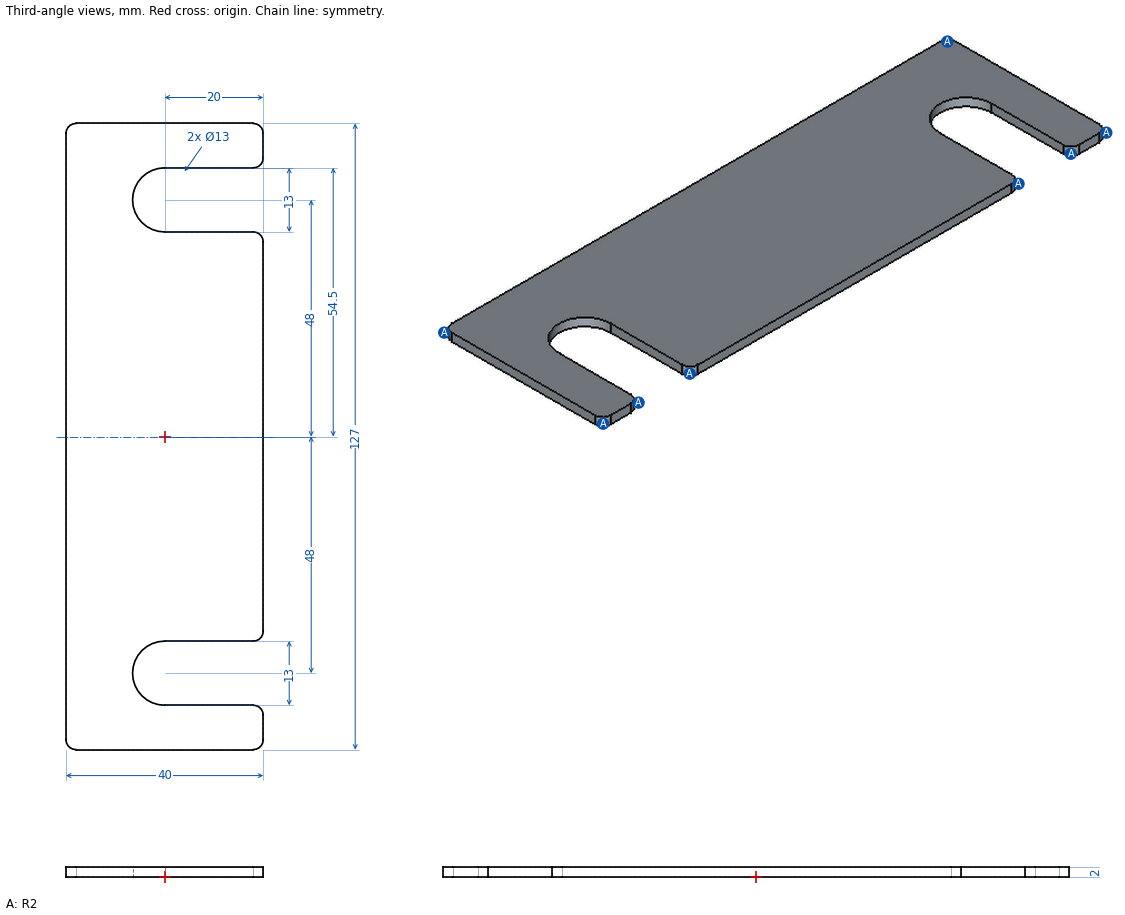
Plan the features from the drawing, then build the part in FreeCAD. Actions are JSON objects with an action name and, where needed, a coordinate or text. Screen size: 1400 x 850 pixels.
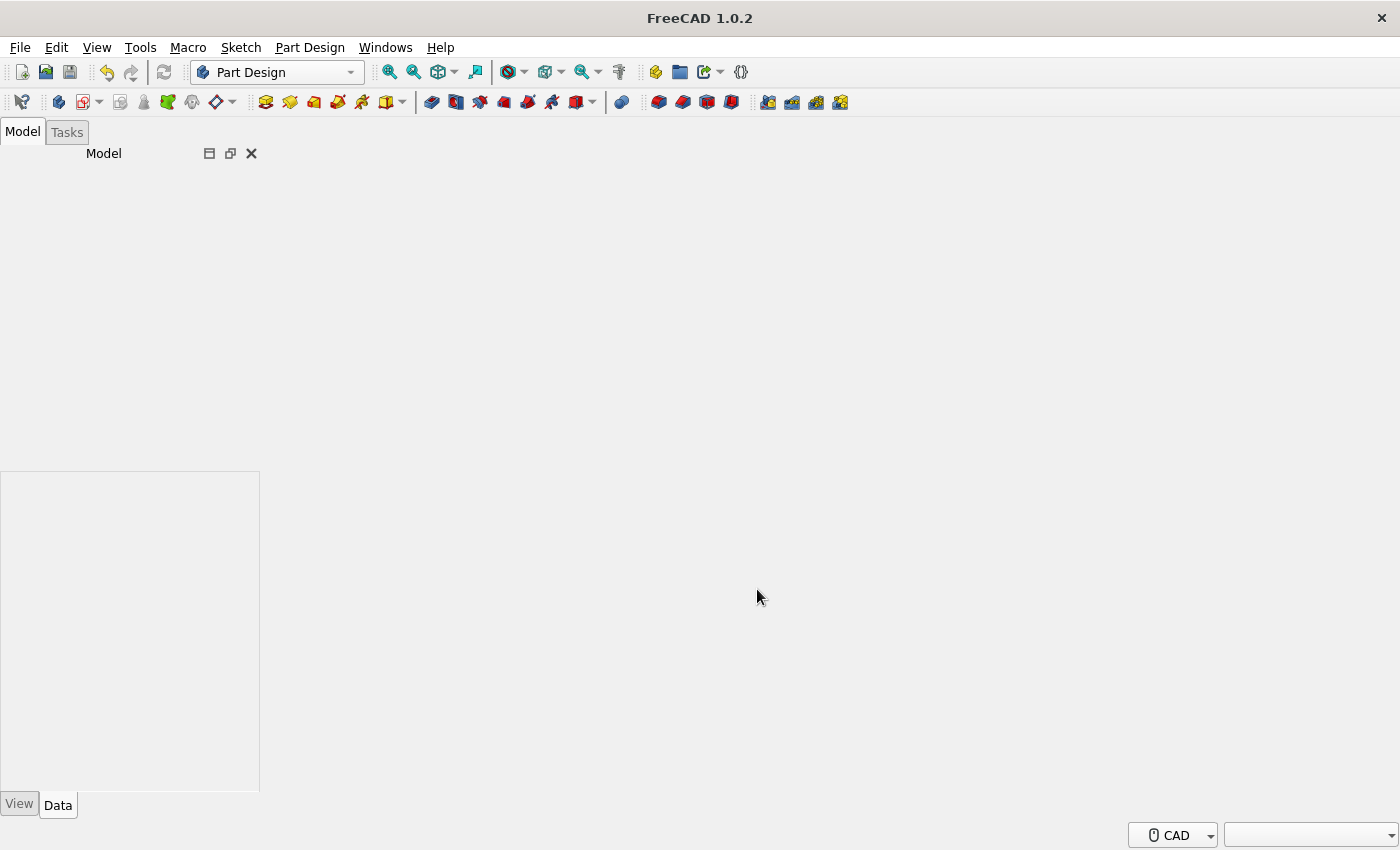
{"action": "left_click", "coordinate": [22, 72]}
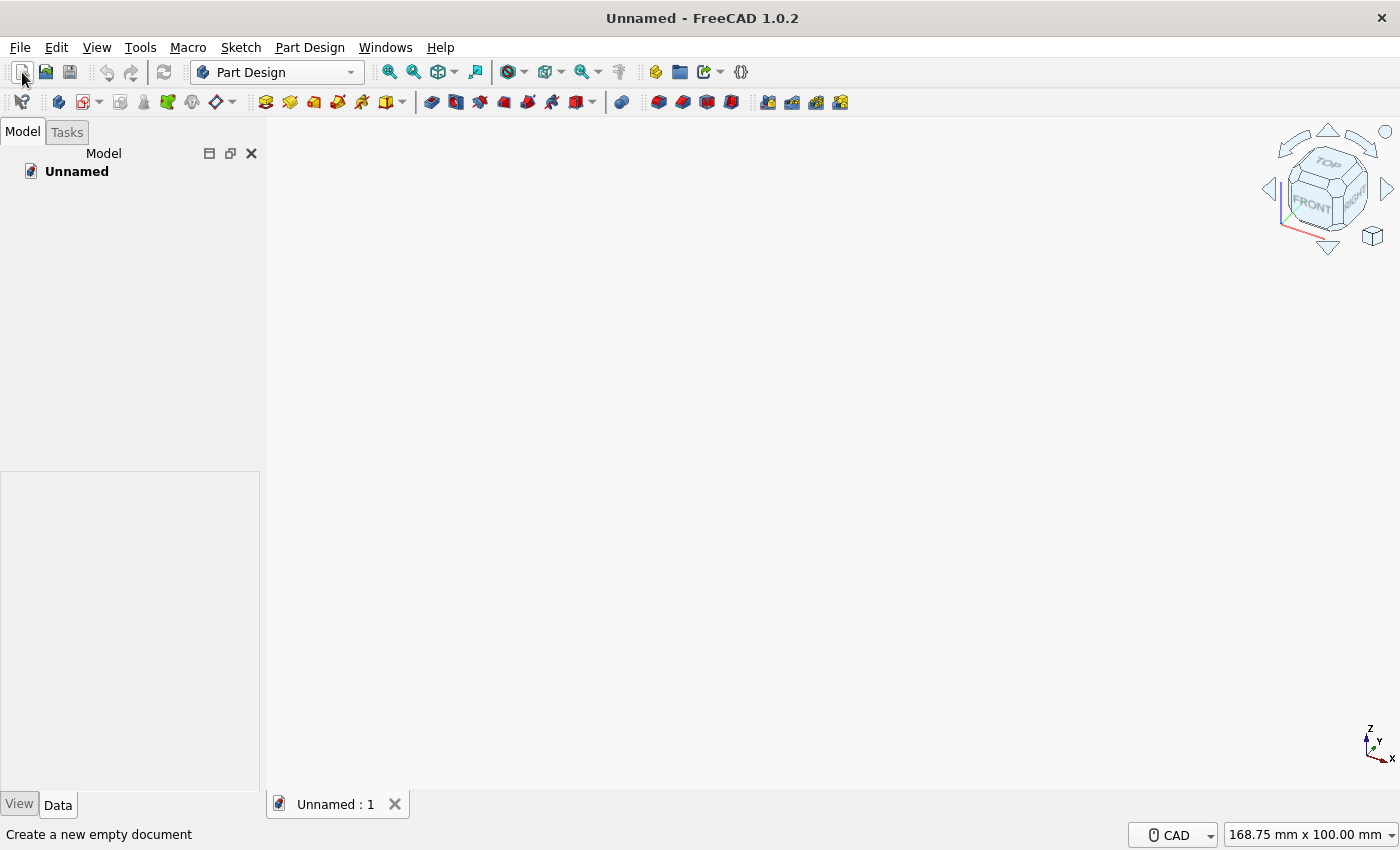
{"action": "left_click", "coordinate": [84, 102]}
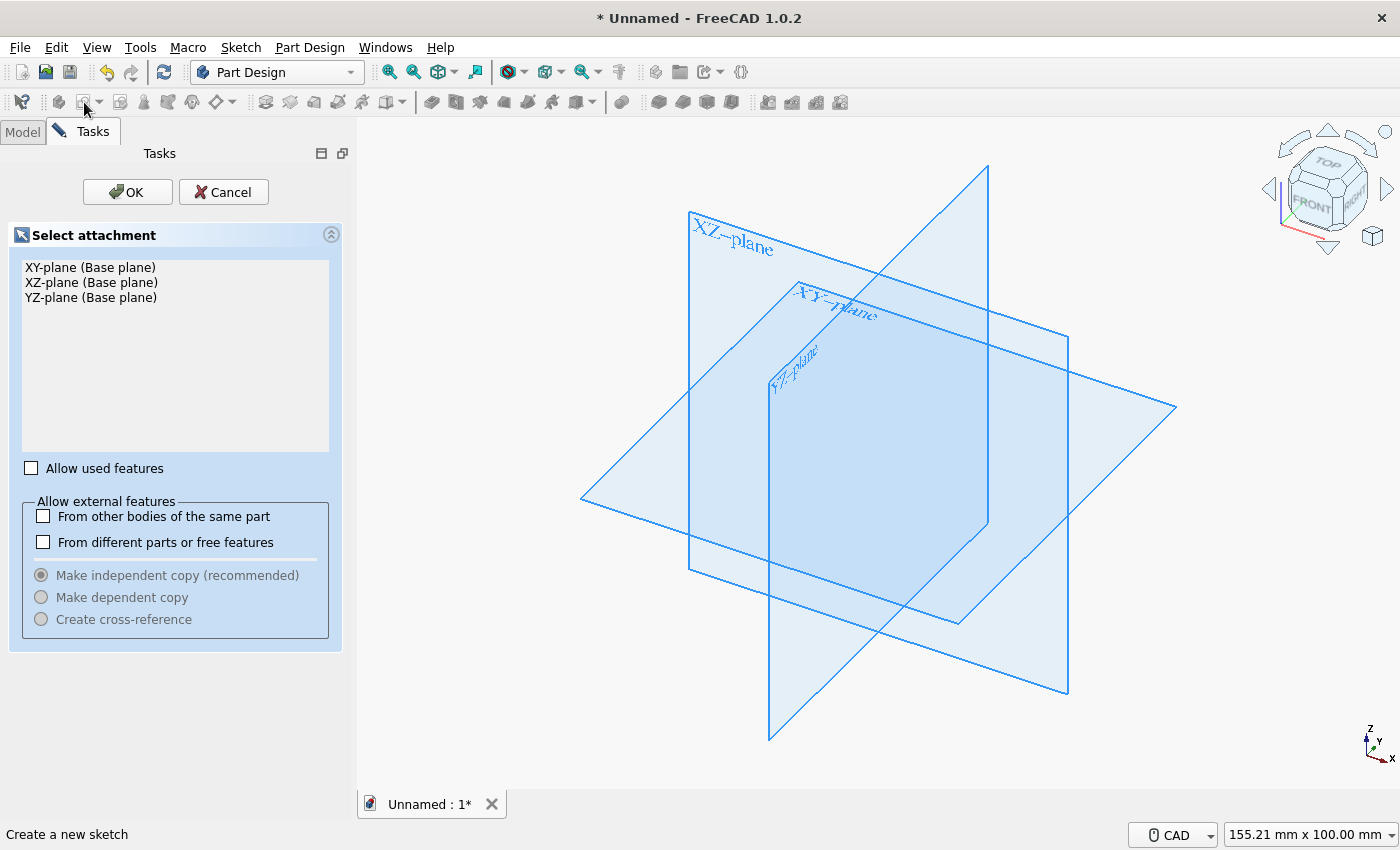
{"action": "left_click", "coordinate": [82, 268]}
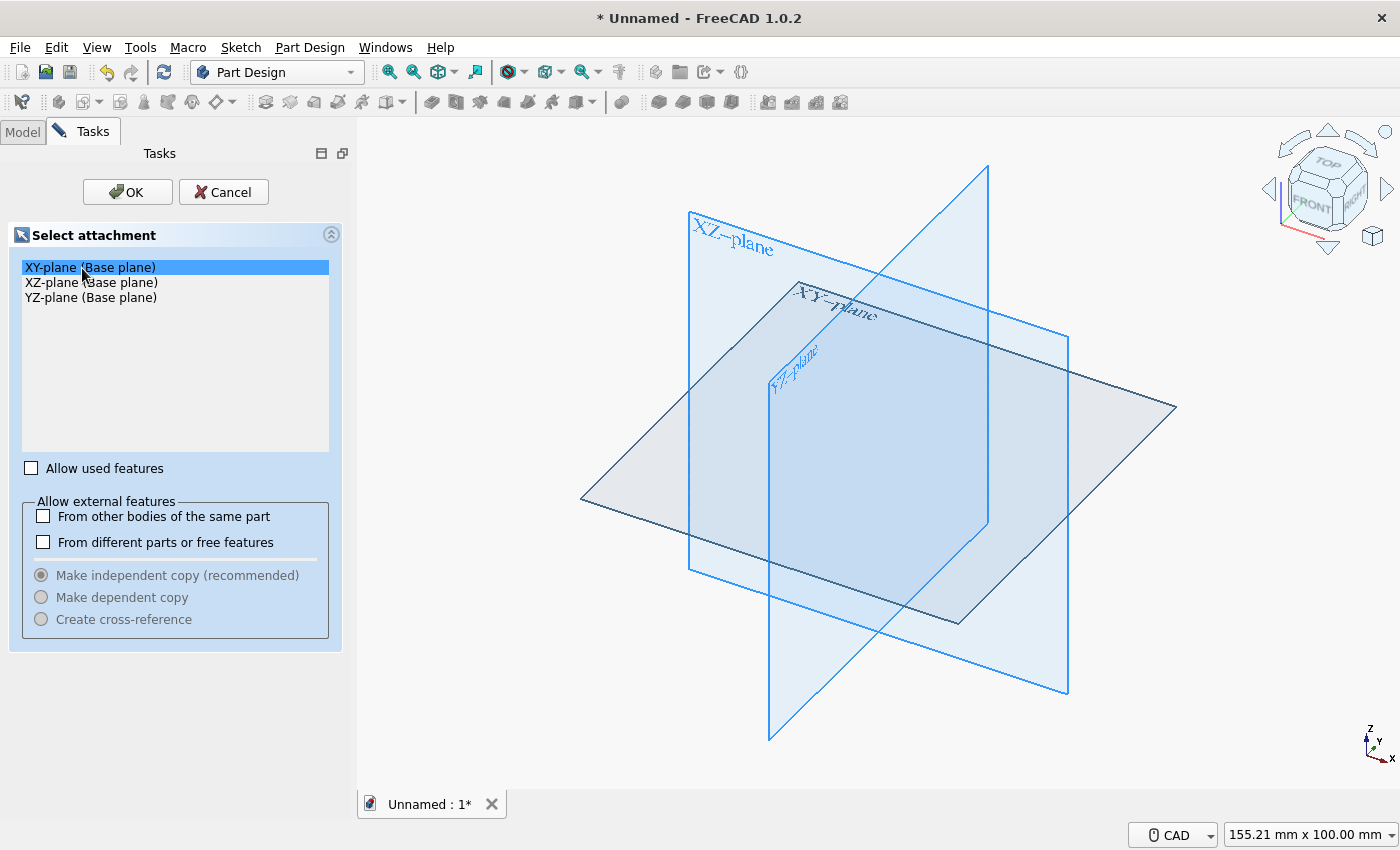
{"action": "left_click", "coordinate": [128, 192]}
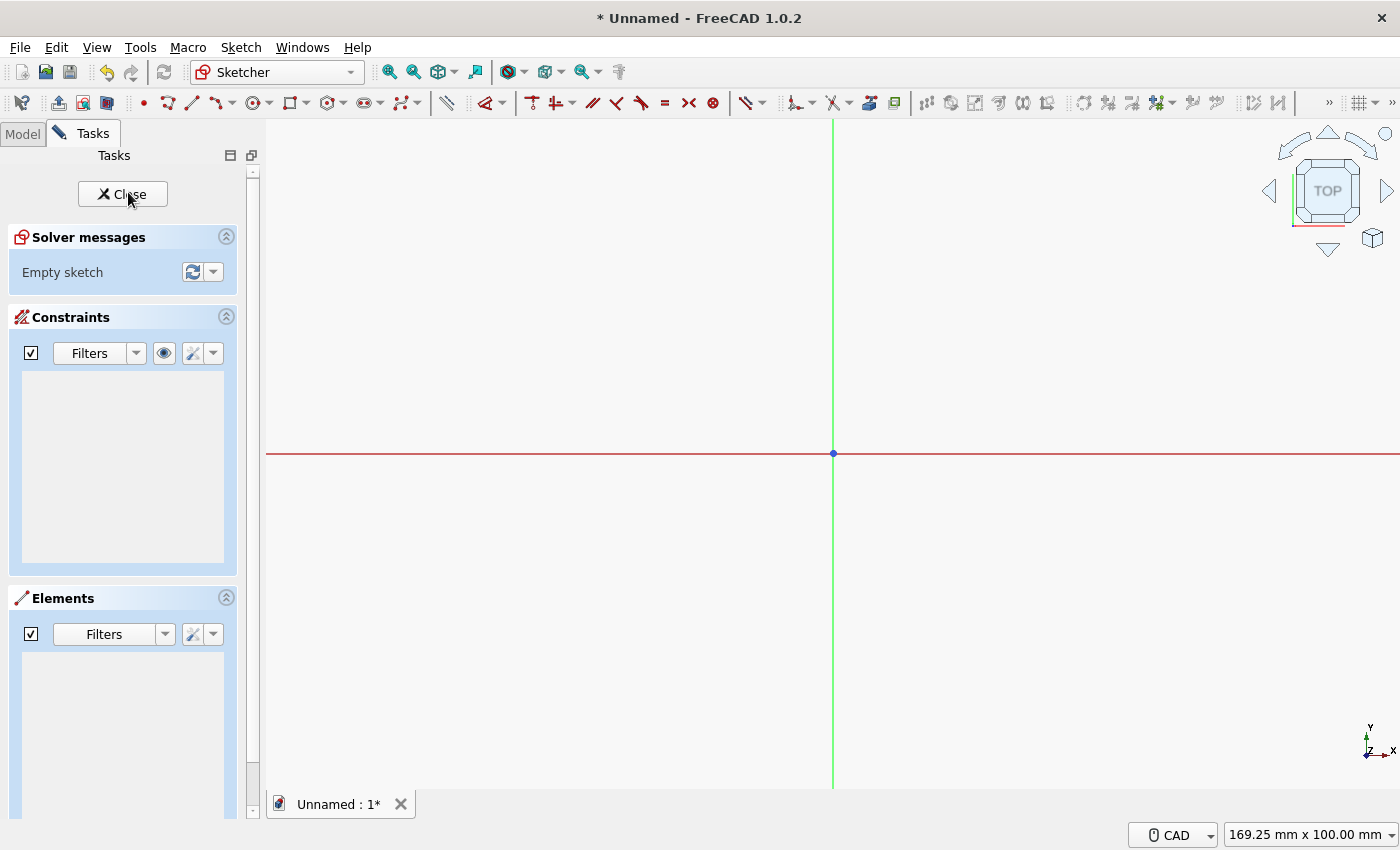
{"action": "scroll", "coordinate": [681, 454], "scroll_direction": "down", "scroll_amount": 3}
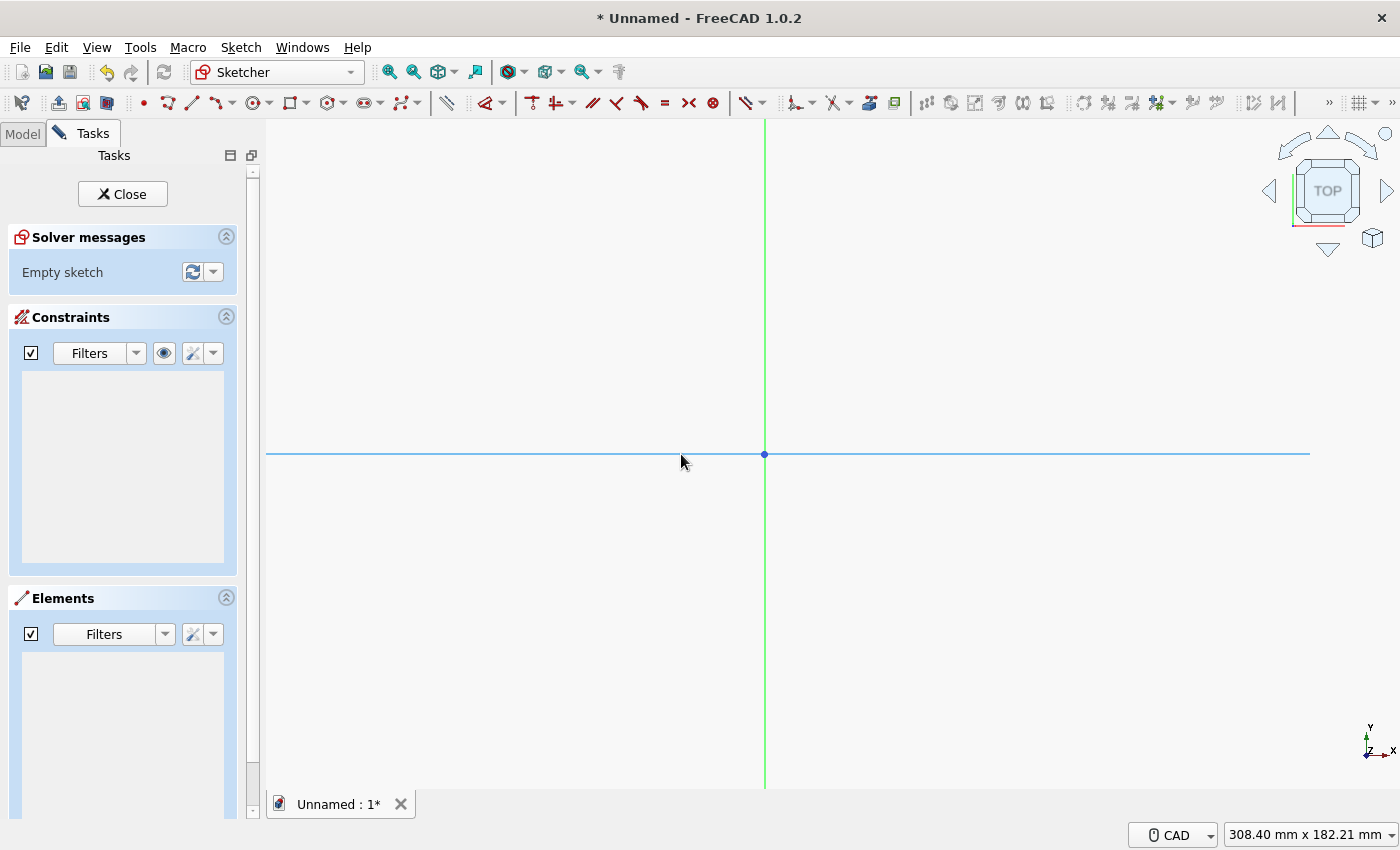
{"action": "key", "text": "g v"}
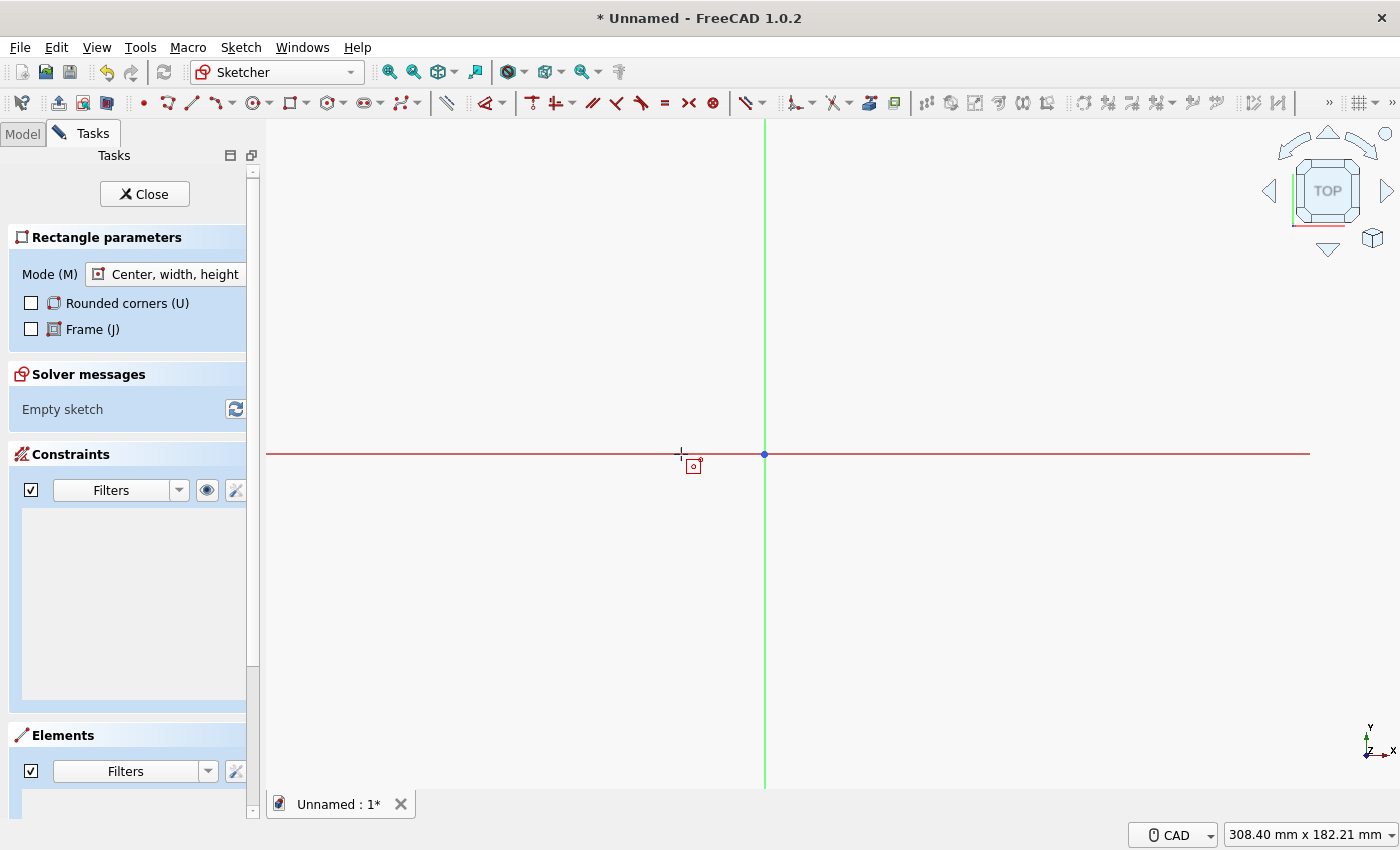
{"action": "left_click", "coordinate": [765, 454]}
{"action": "left_click", "coordinate": [838, 221]}
{"action": "key", "text": "Escape"}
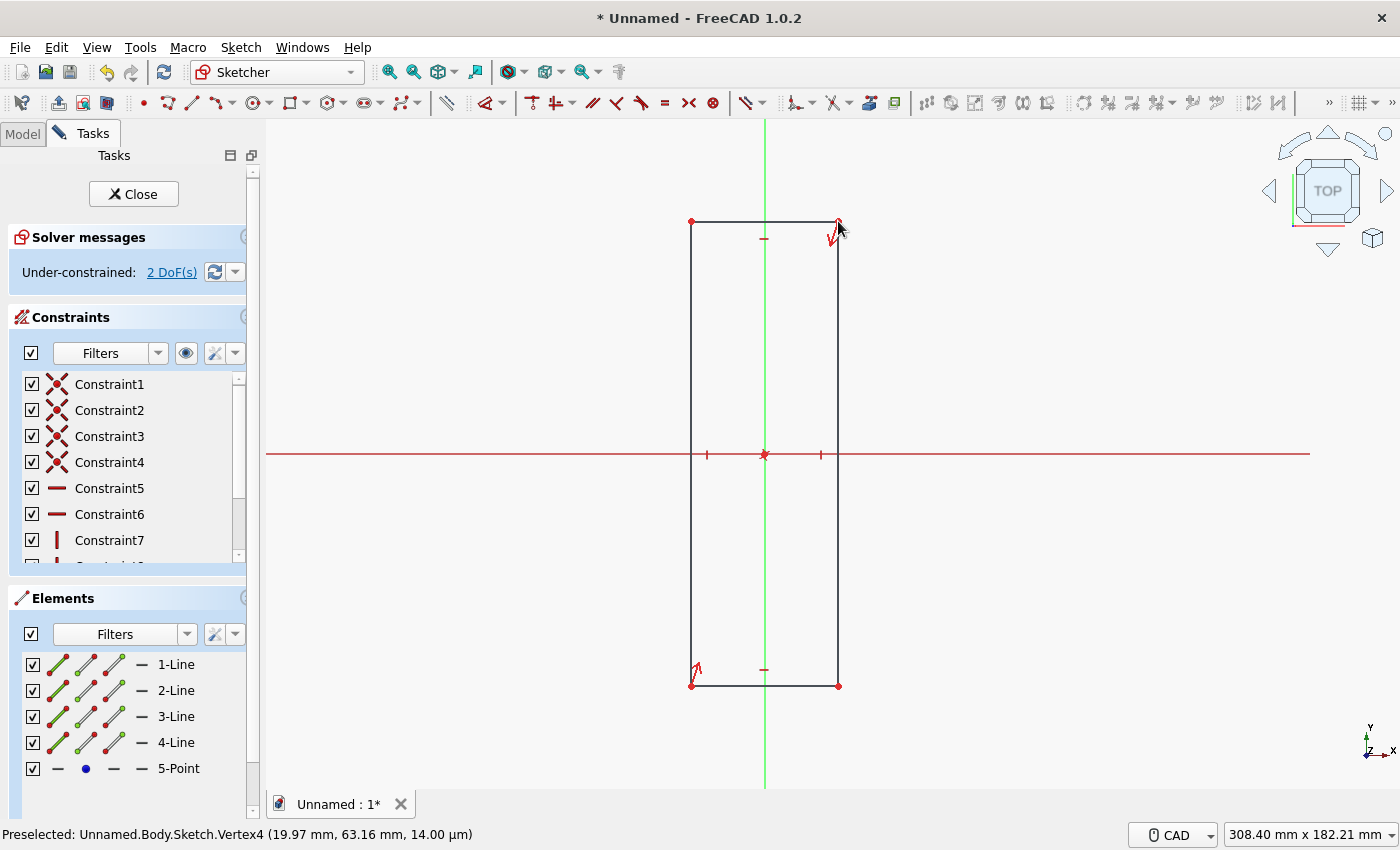
{"action": "left_click", "coordinate": [486, 104]}